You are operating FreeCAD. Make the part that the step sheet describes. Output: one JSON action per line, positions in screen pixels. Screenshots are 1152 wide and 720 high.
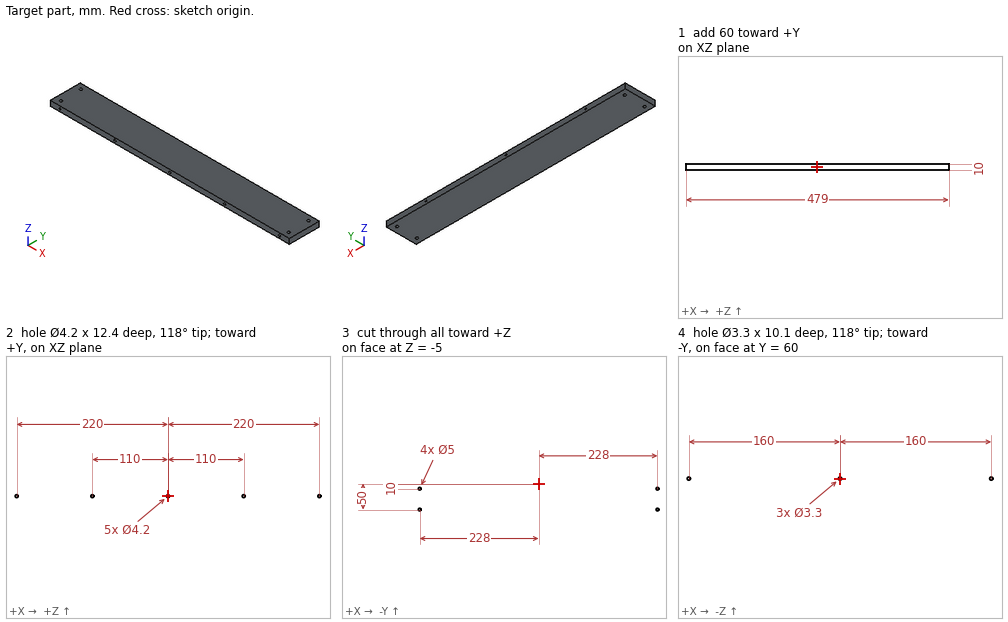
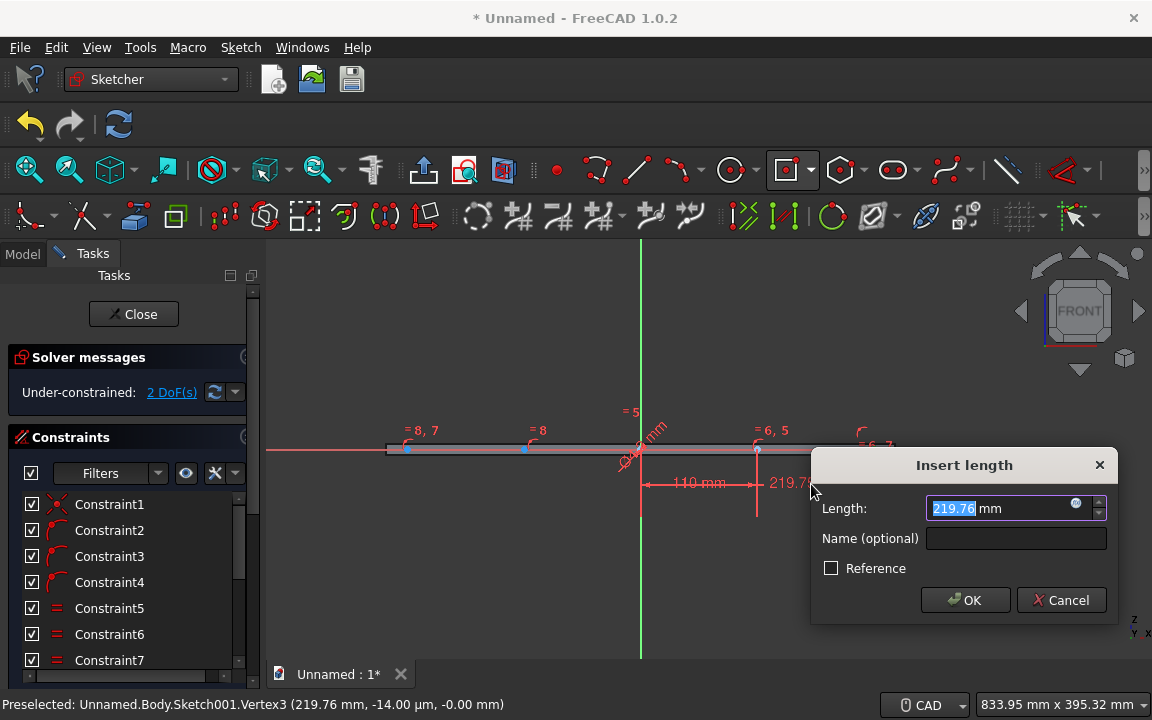
{"action": "type", "text": "220"}
{"action": "key", "text": "Return"}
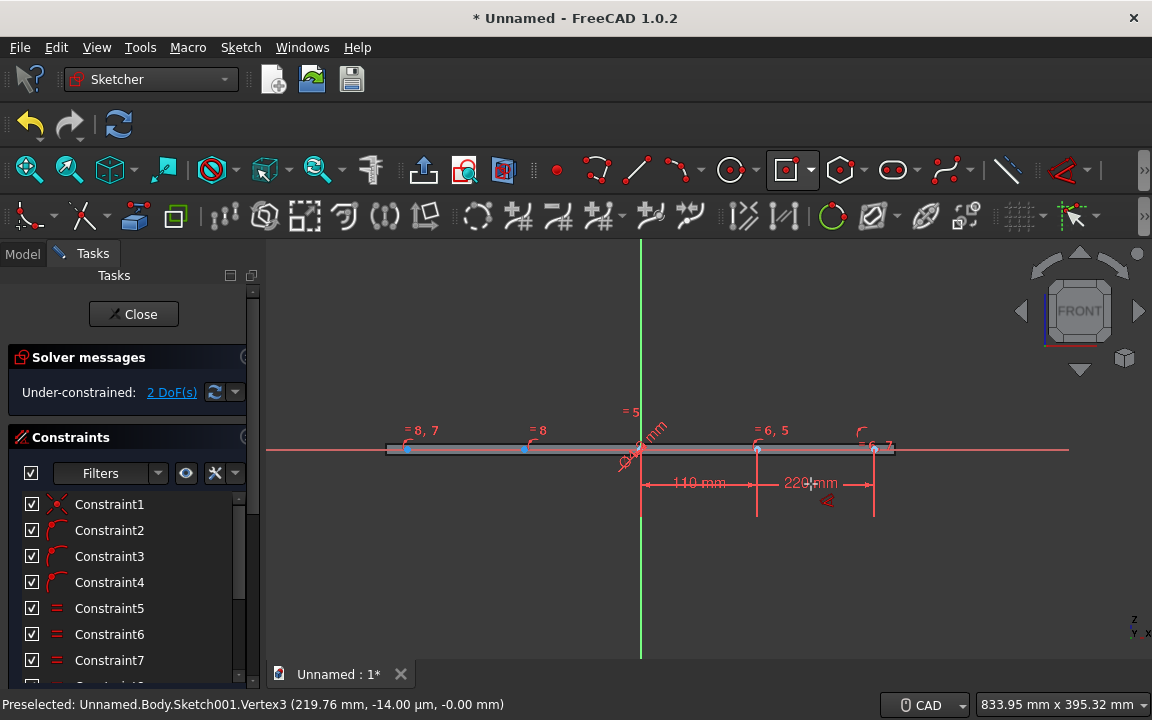
{"action": "left_click", "coordinate": [407, 450]}
{"action": "left_click", "coordinate": [524, 484]}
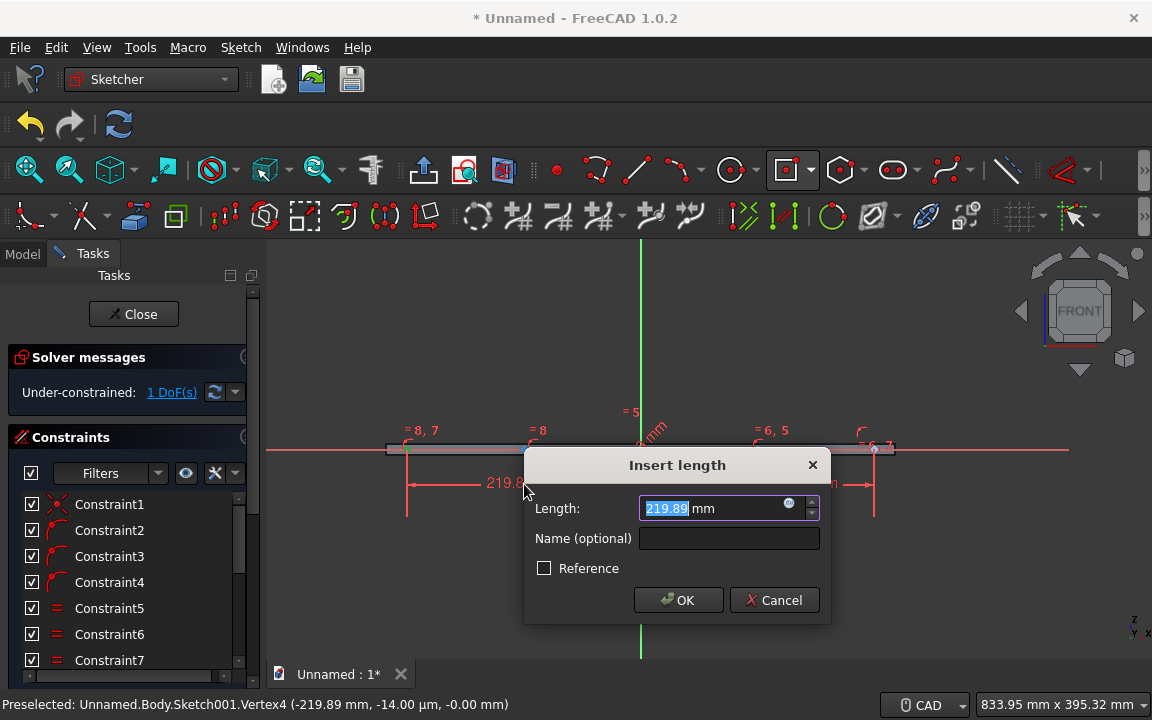
{"action": "type", "text": "220"}
{"action": "key", "text": "Return"}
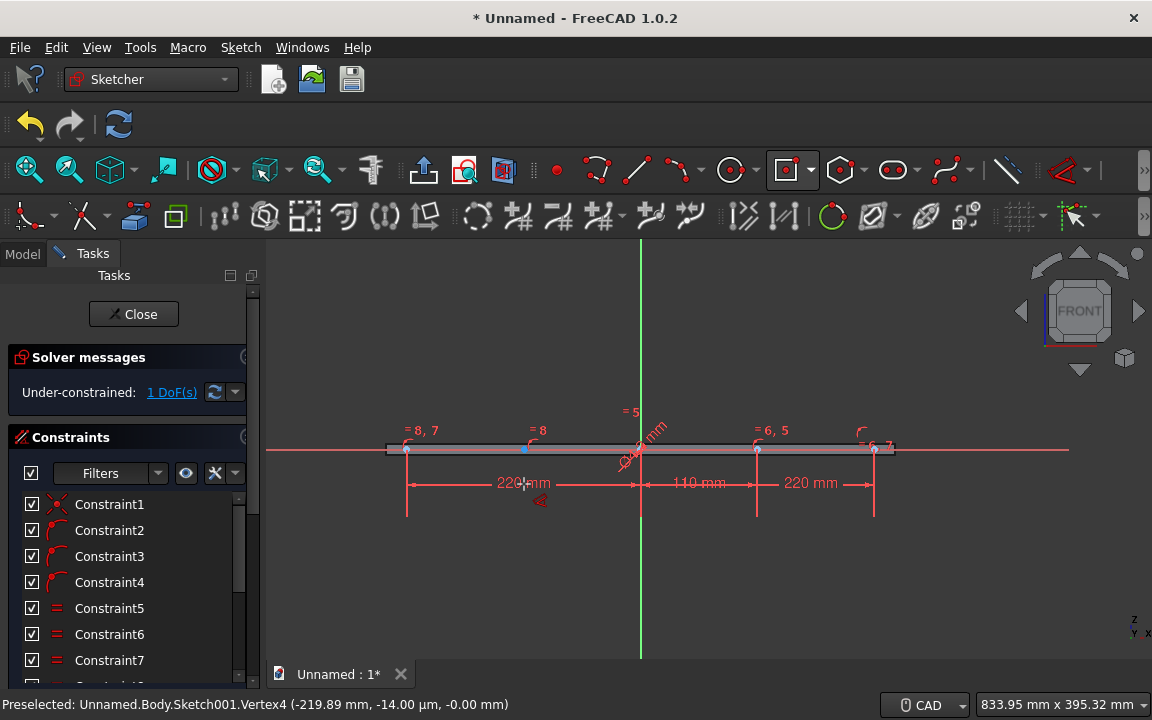
{"action": "left_click", "coordinate": [524, 450]}
{"action": "left_click", "coordinate": [609, 484]}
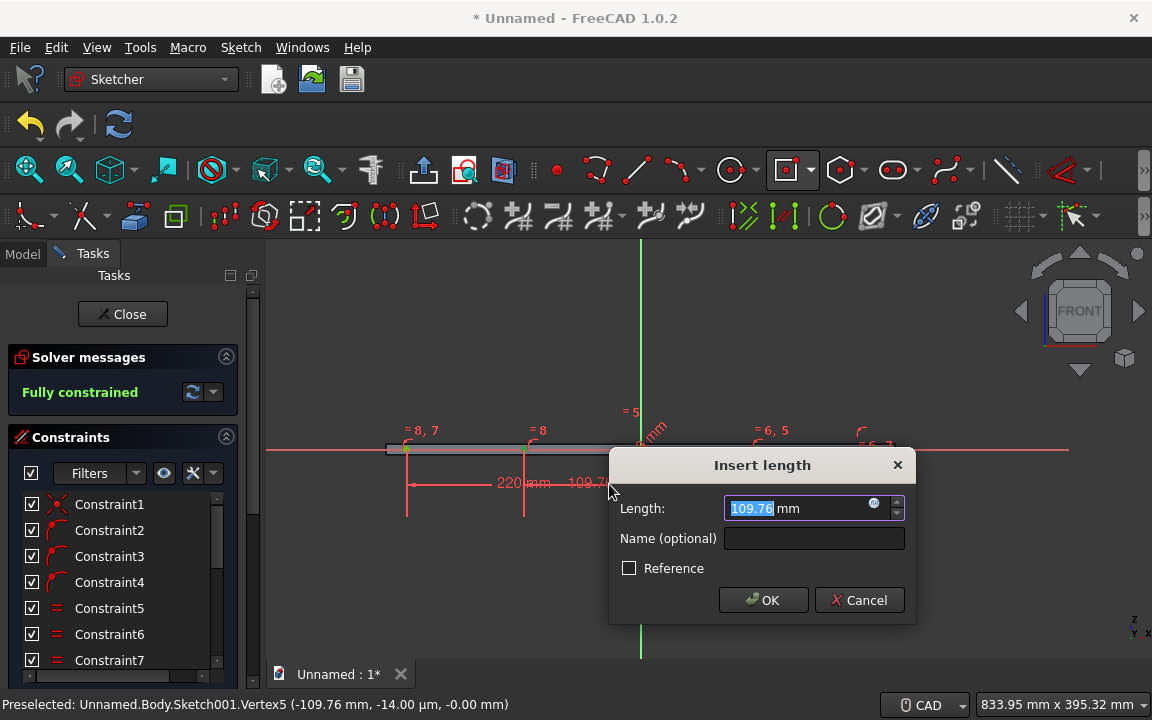
{"action": "type", "text": "110"}
{"action": "key", "text": "Return"}
{"action": "key", "text": "Escape"}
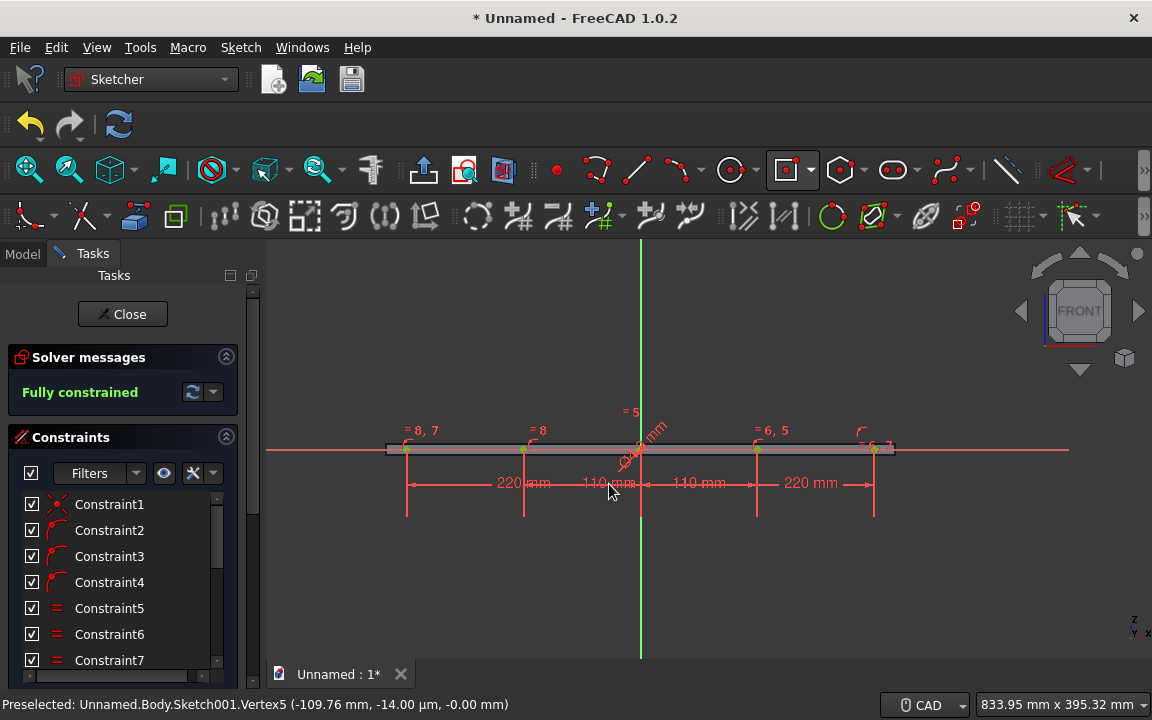
{"action": "left_click", "coordinate": [123, 314]}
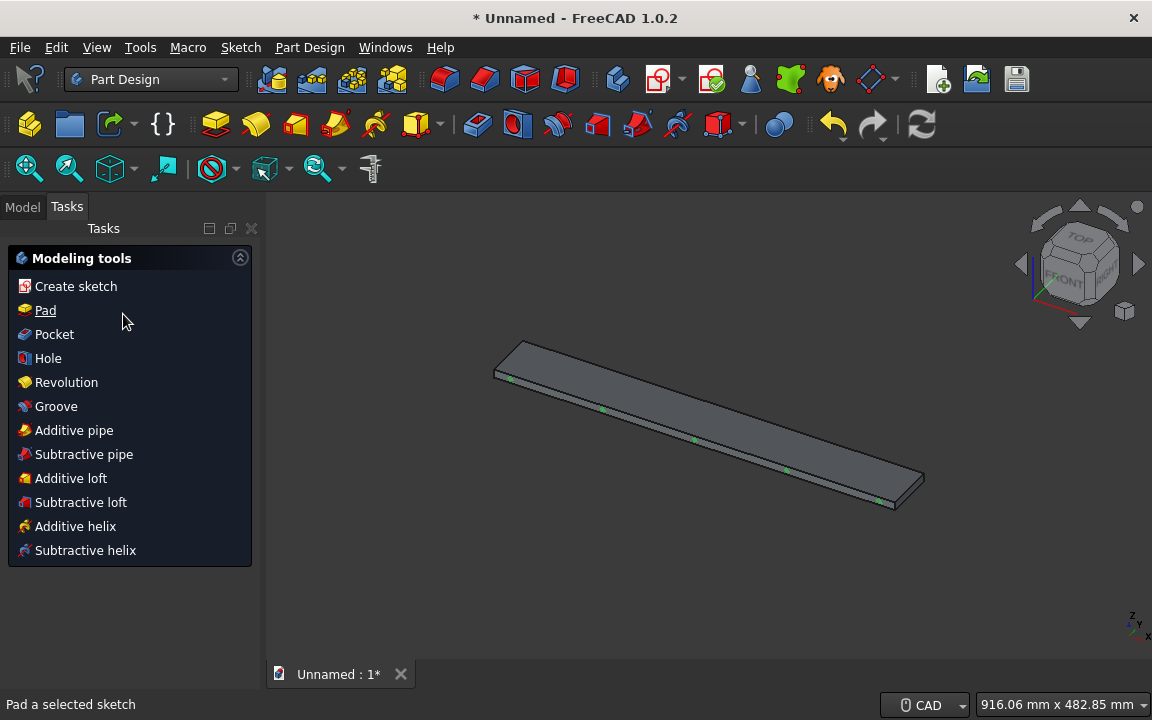
{"action": "left_click", "coordinate": [518, 124]}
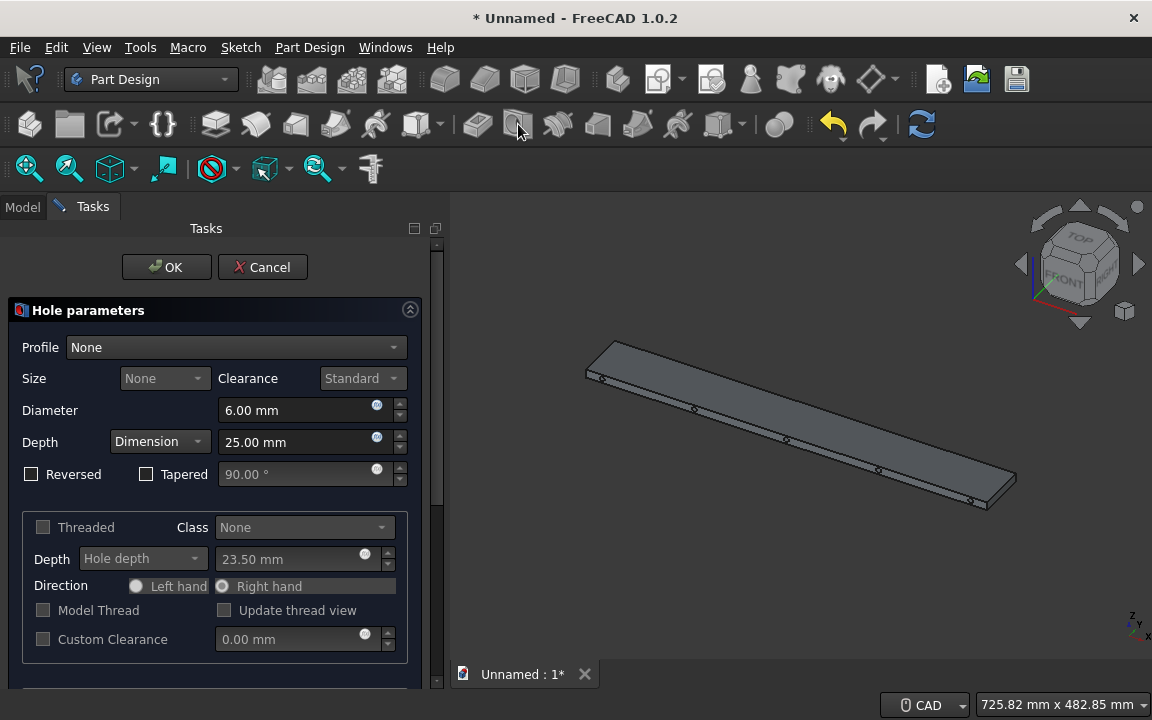
{"action": "triple_click", "coordinate": [305, 410]}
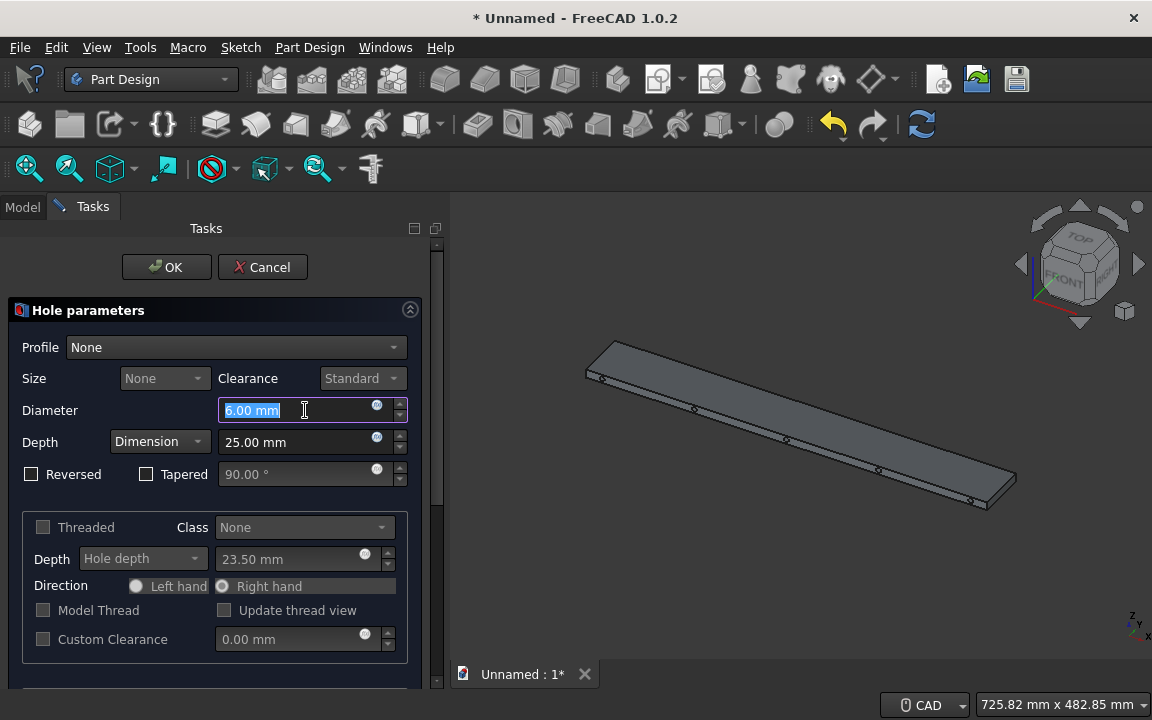
{"action": "type", "text": "4.2"}
{"action": "key", "text": "Tab"}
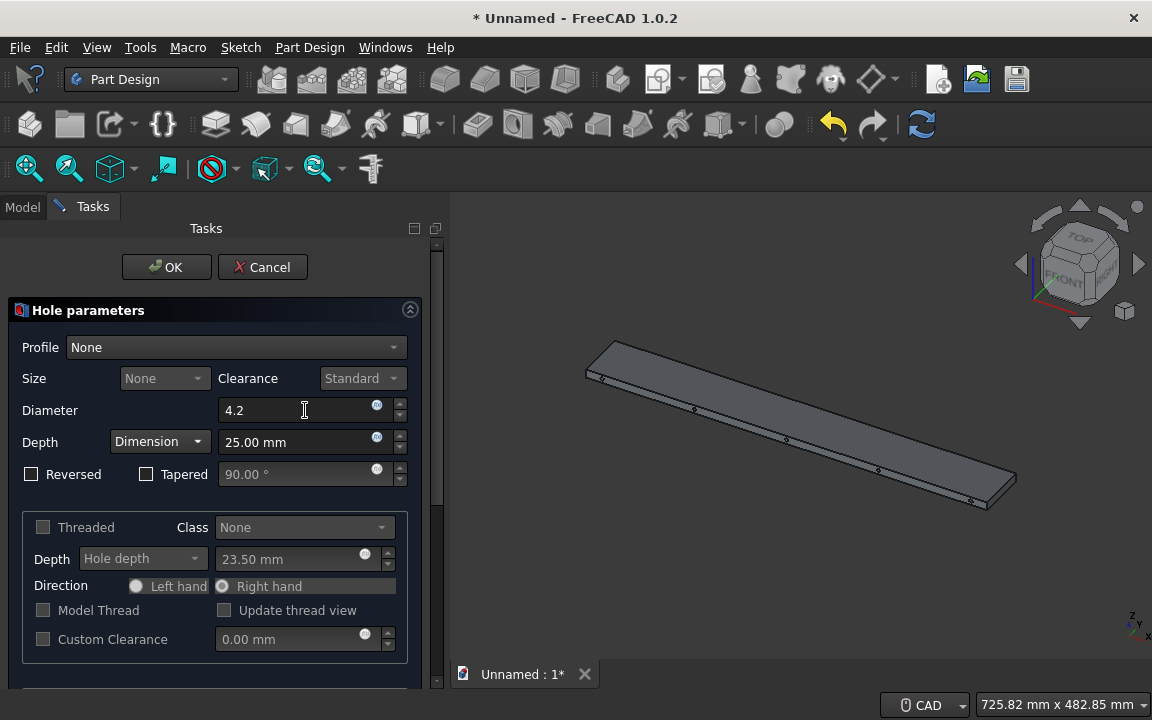
{"action": "triple_click", "coordinate": [305, 442]}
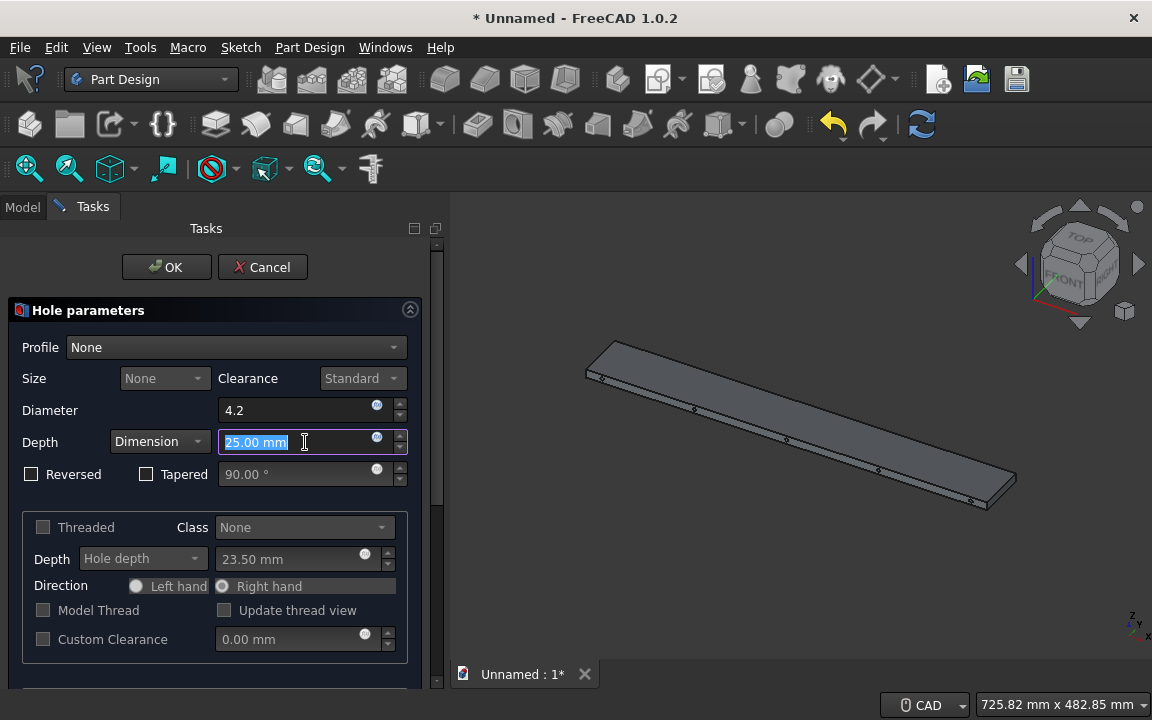
{"action": "type", "text": "12.4"}
{"action": "key", "text": "Tab"}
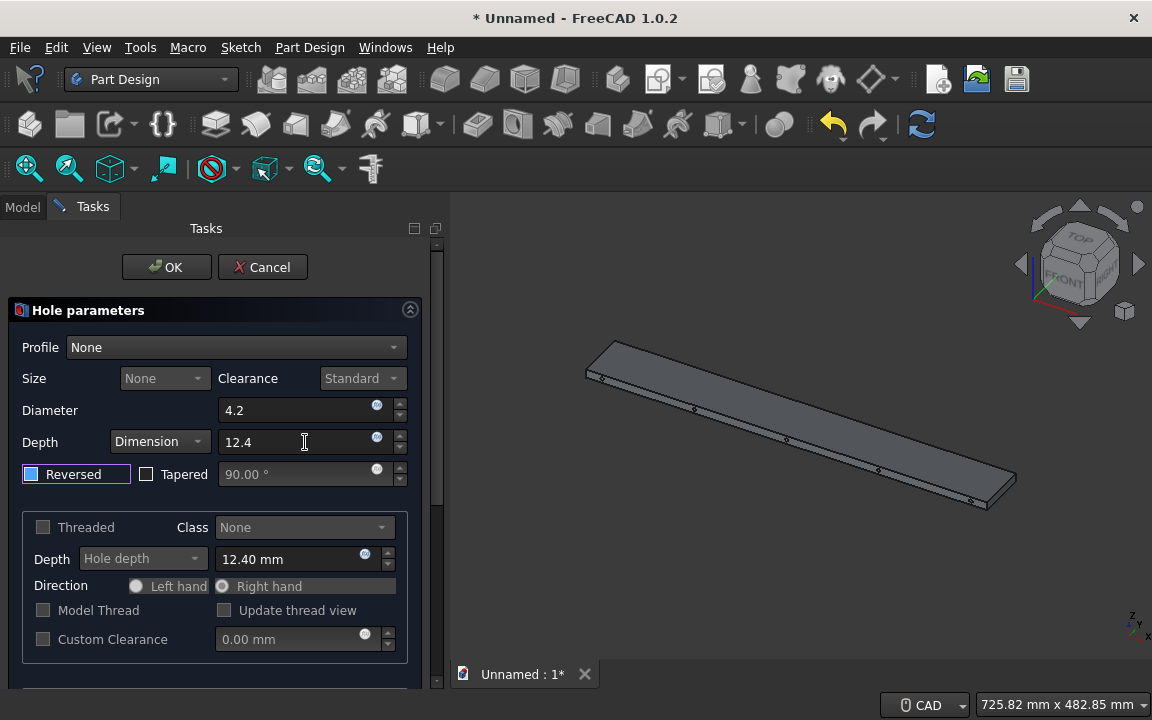
{"action": "left_click", "coordinate": [167, 267]}